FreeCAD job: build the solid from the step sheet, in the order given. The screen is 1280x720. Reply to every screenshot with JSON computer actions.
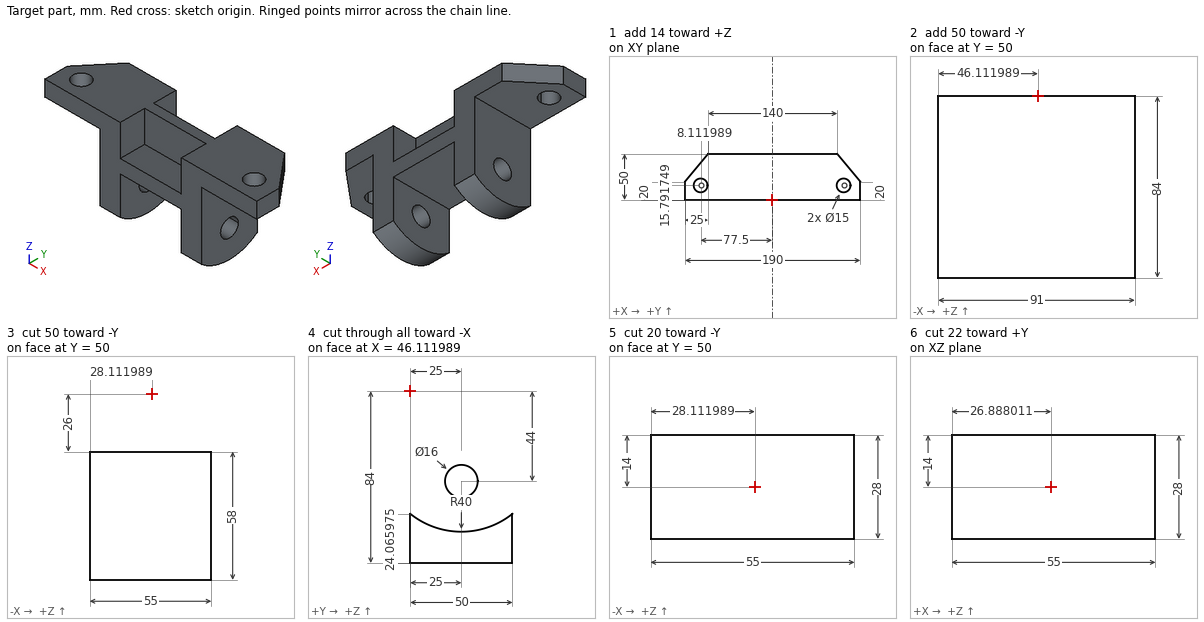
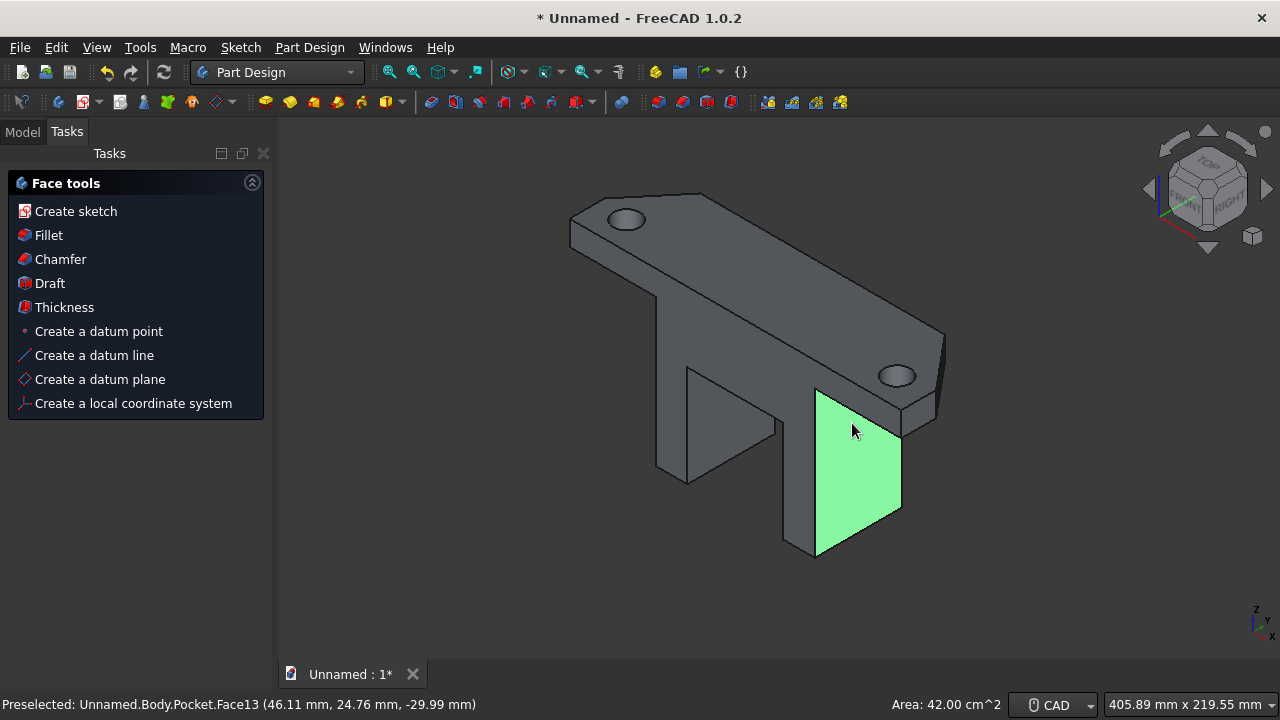
{"action": "left_click", "coordinate": [84, 102]}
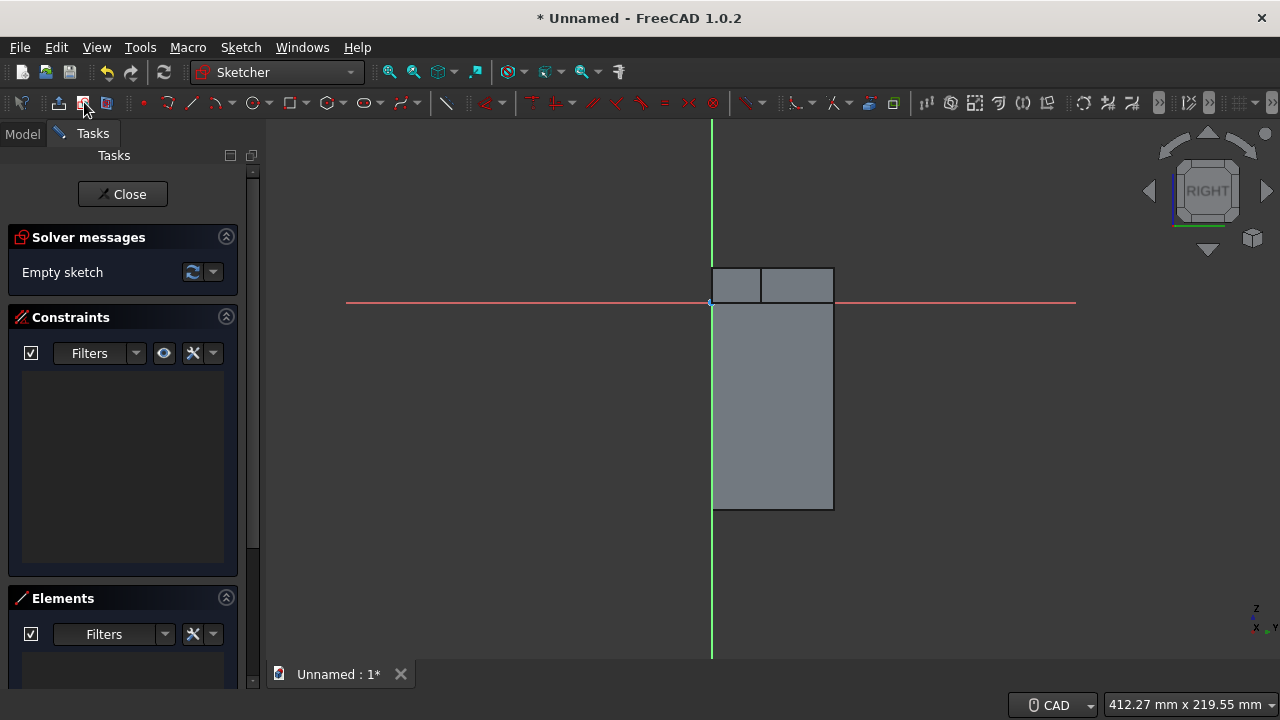
{"action": "left_click", "coordinate": [108, 104]}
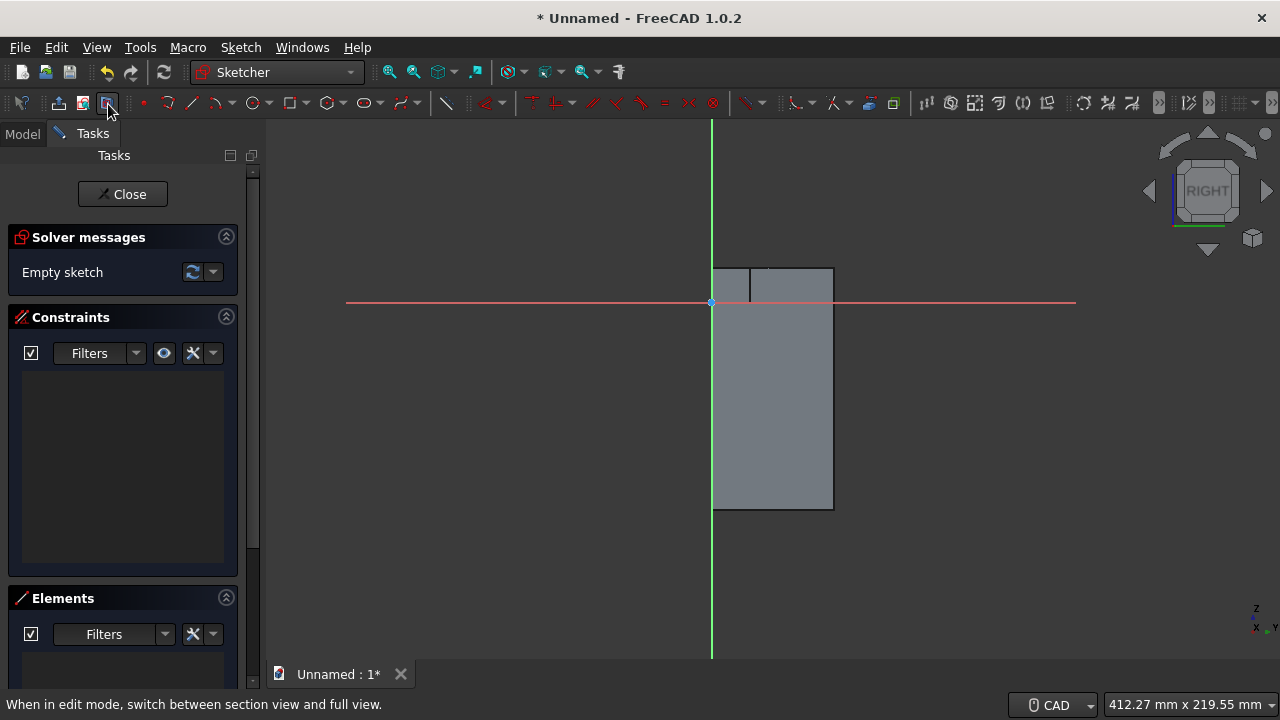
{"action": "scroll", "coordinate": [856, 427], "scroll_direction": "up", "scroll_amount": 3}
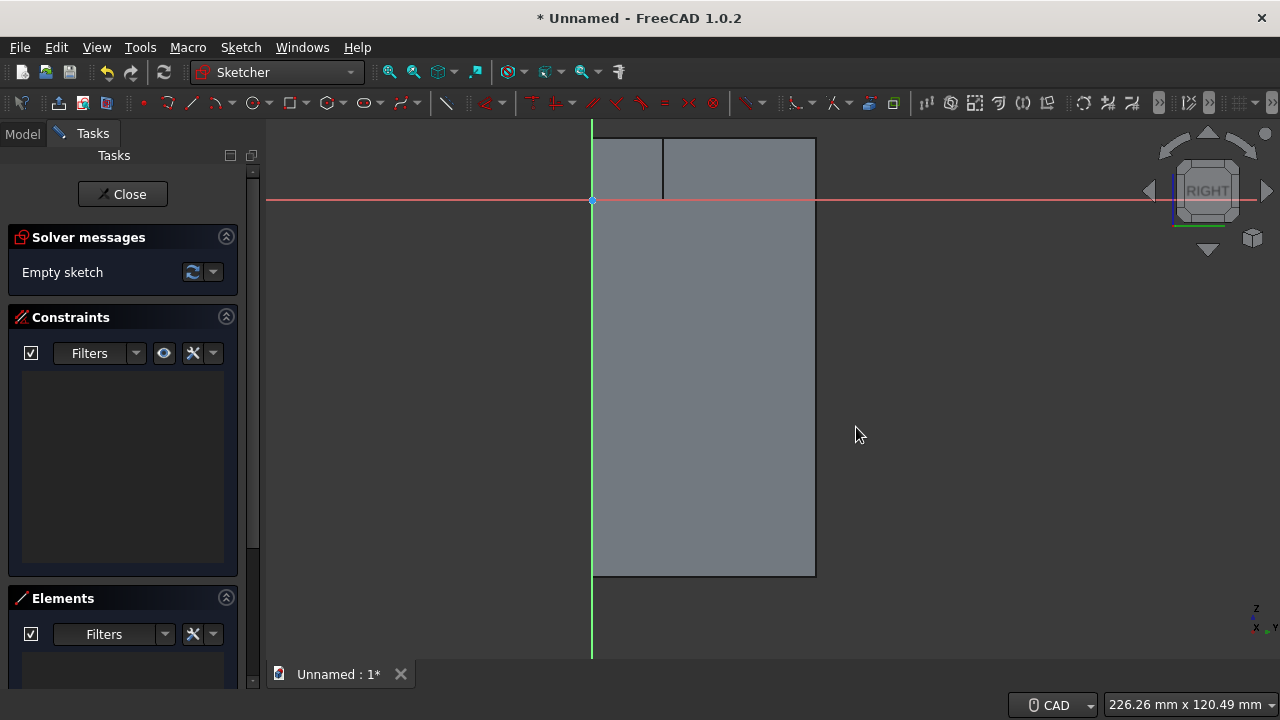
{"action": "left_click", "coordinate": [168, 104]}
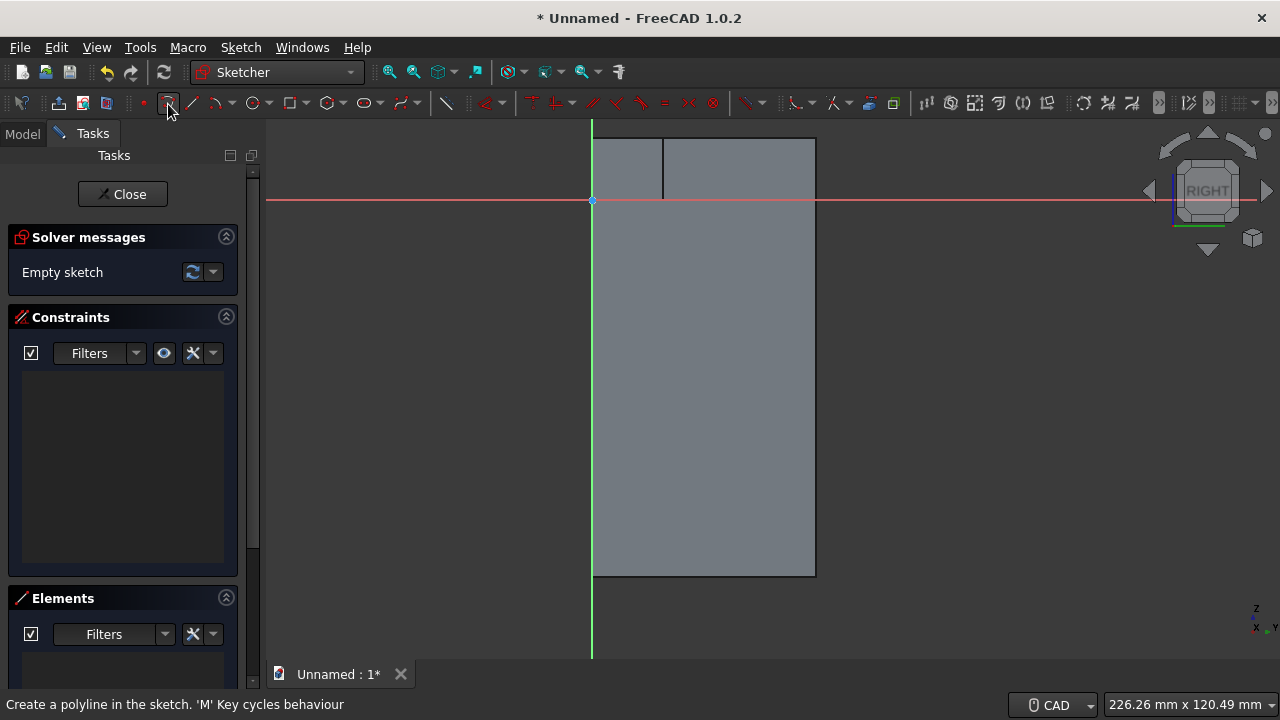
{"action": "left_click", "coordinate": [592, 469]}
{"action": "left_click", "coordinate": [601, 577]}
{"action": "left_click", "coordinate": [816, 577]}
{"action": "left_click", "coordinate": [816, 469]}
{"action": "right_click", "coordinate": [816, 469]}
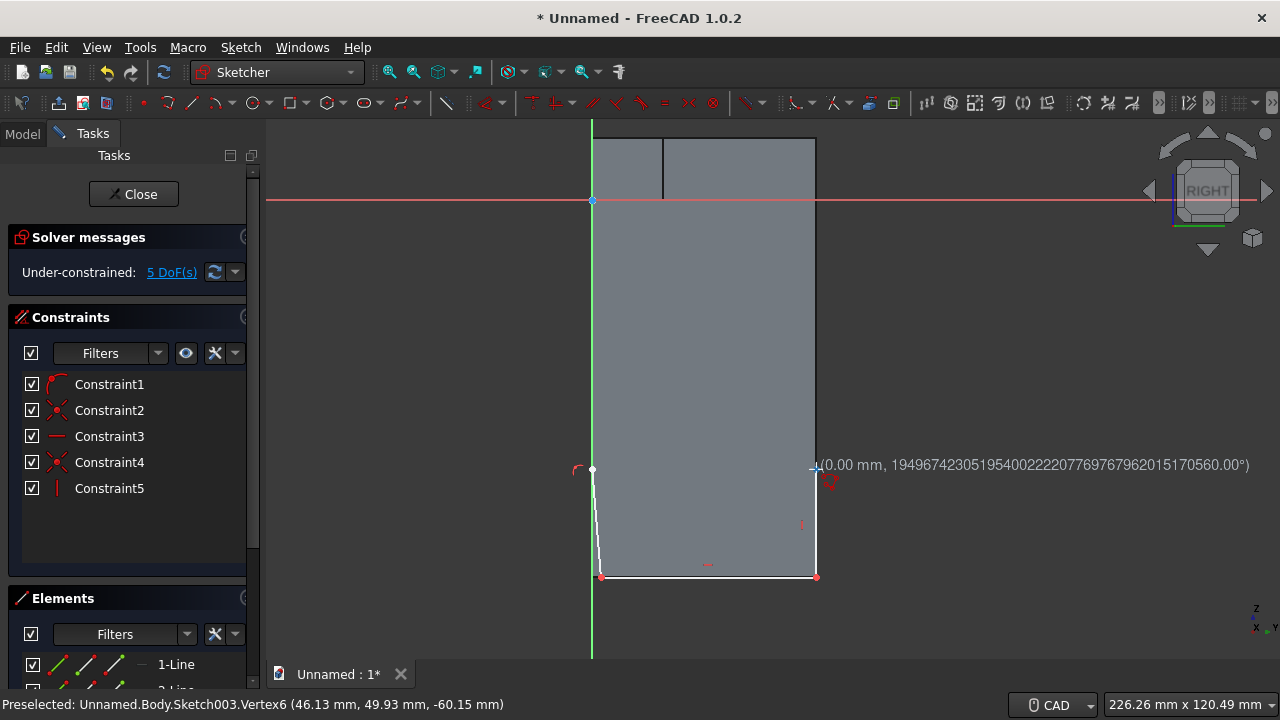
{"action": "left_click", "coordinate": [234, 104]}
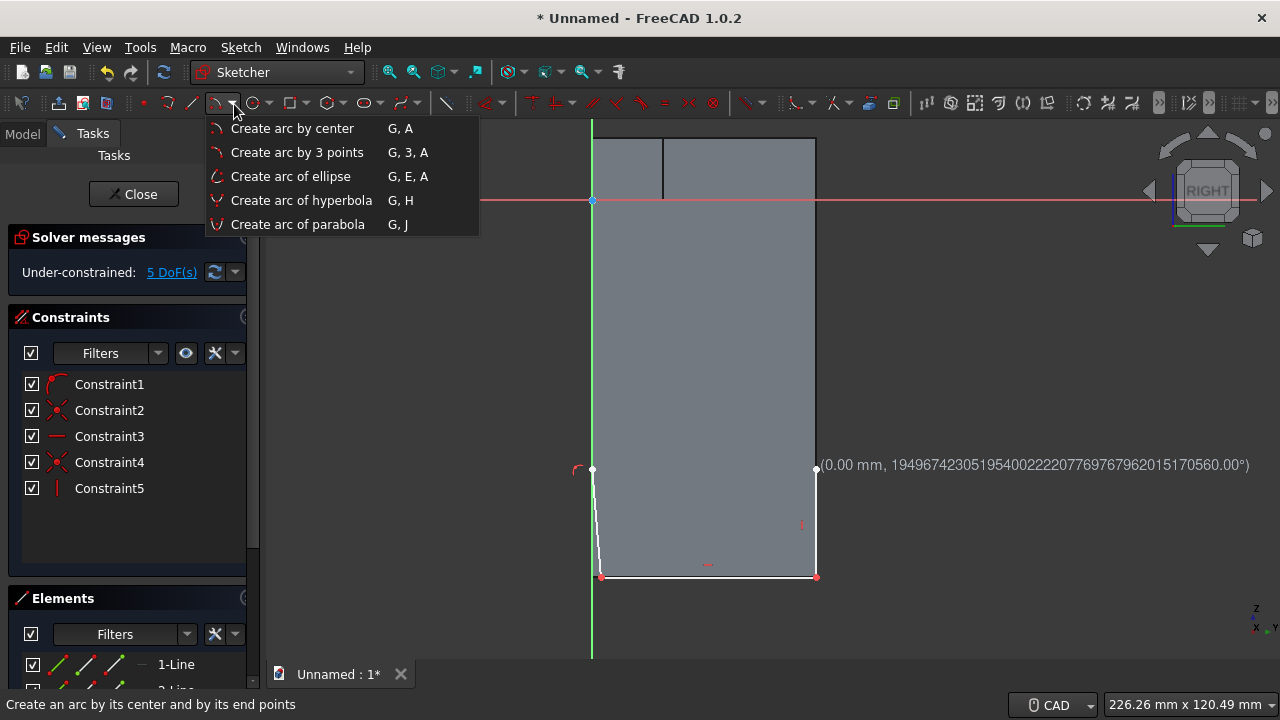
{"action": "left_click", "coordinate": [342, 152]}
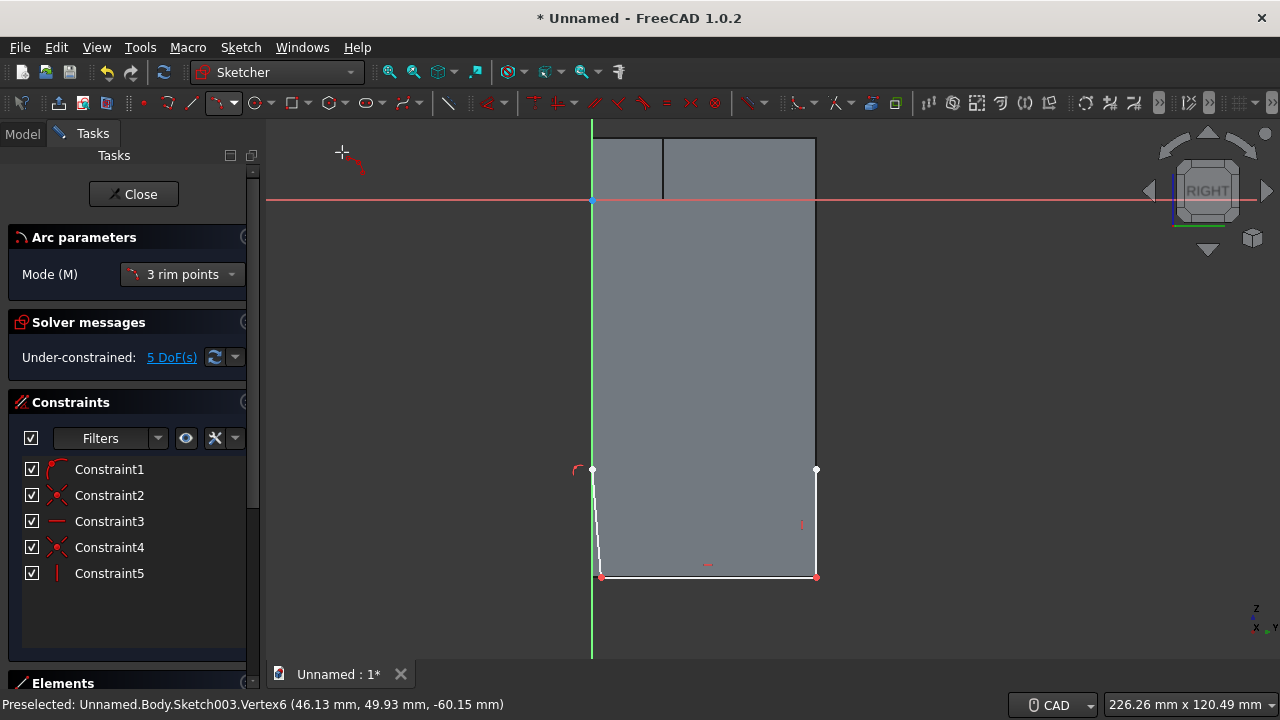
{"action": "left_click", "coordinate": [816, 470]}
{"action": "left_click", "coordinate": [592, 470]}
{"action": "left_click", "coordinate": [704, 508]}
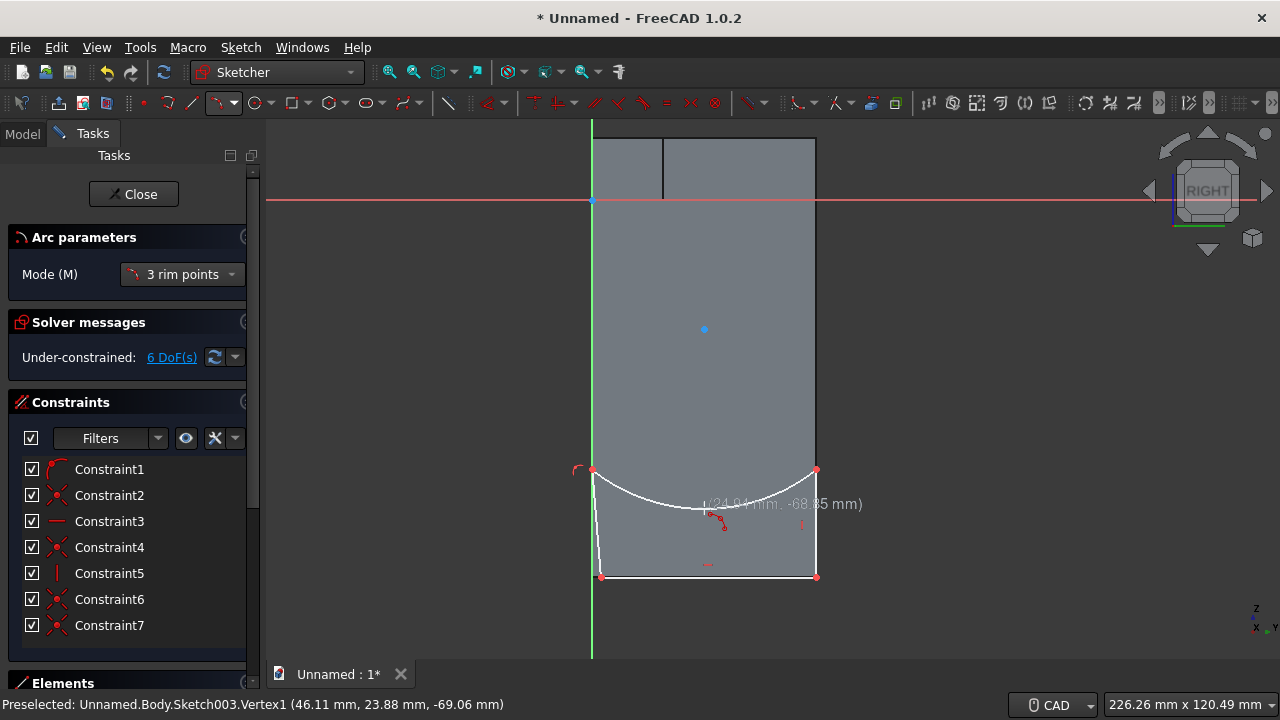
{"action": "left_click", "coordinate": [256, 104]}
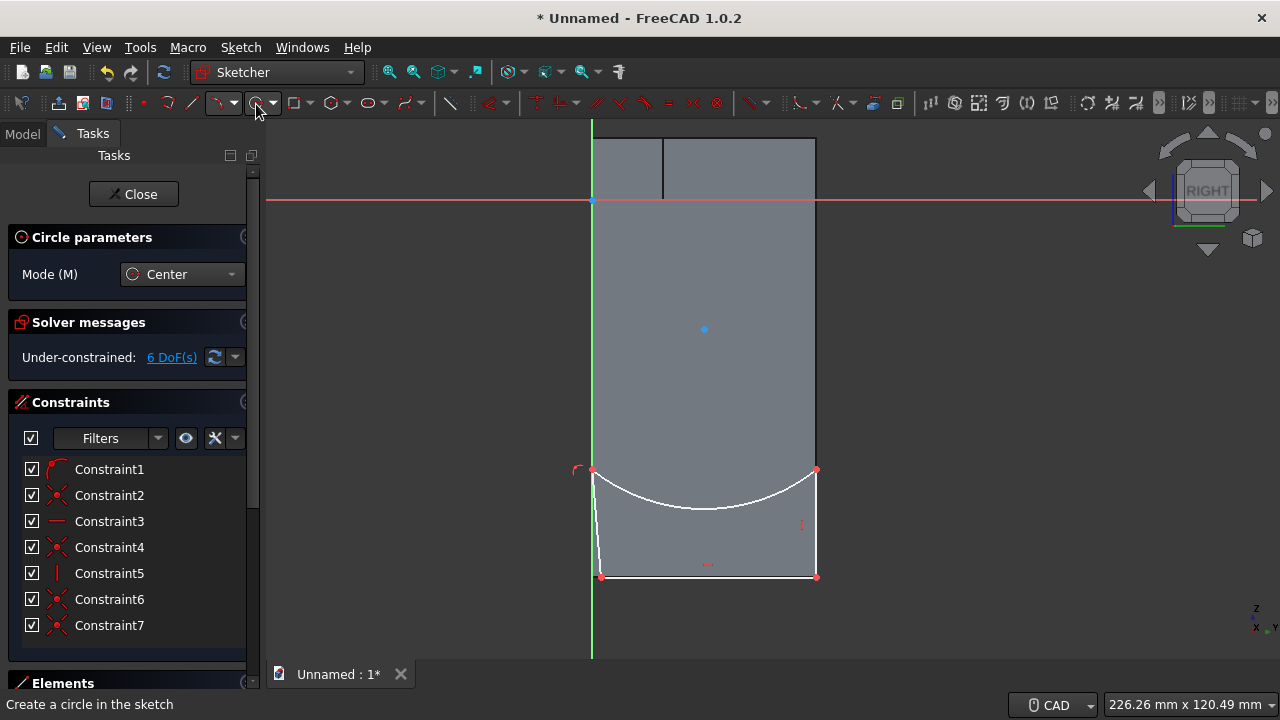
{"action": "left_click", "coordinate": [704, 398]}
{"action": "mouse_move", "coordinate": [730, 372]}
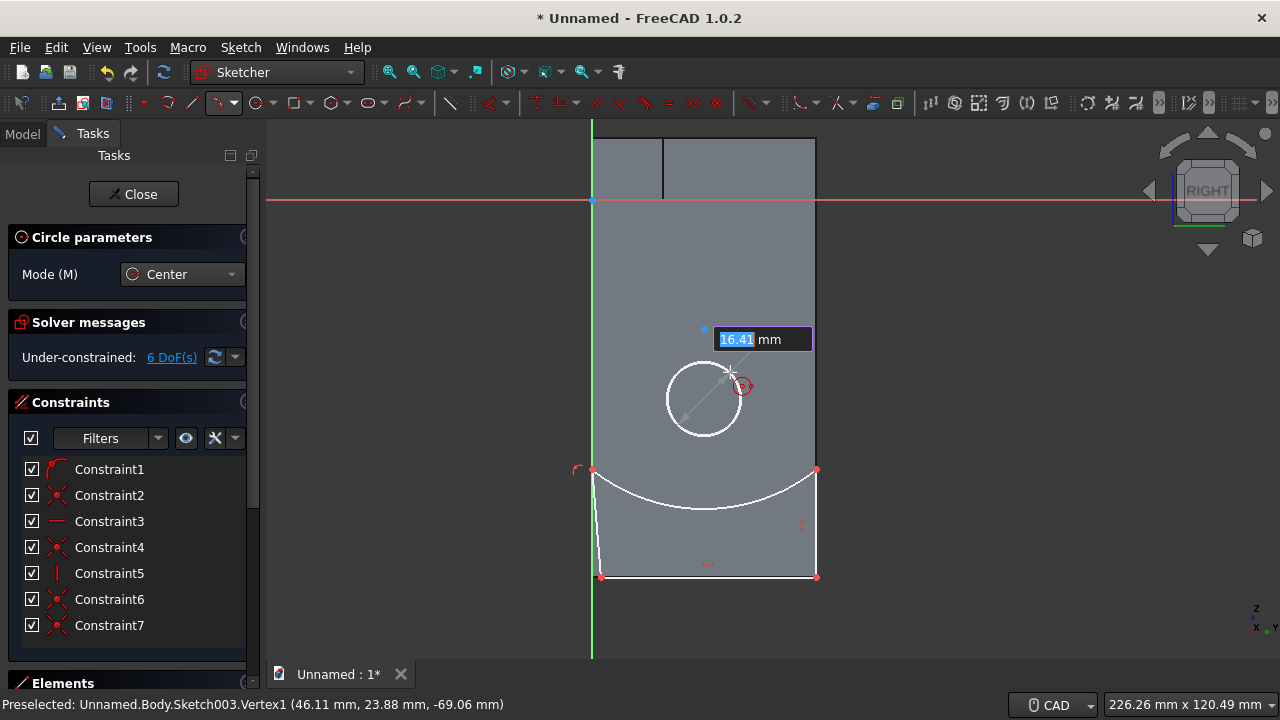
{"action": "type", "text": "16"}
{"action": "key", "text": "Return"}
{"action": "key", "text": "Escape"}